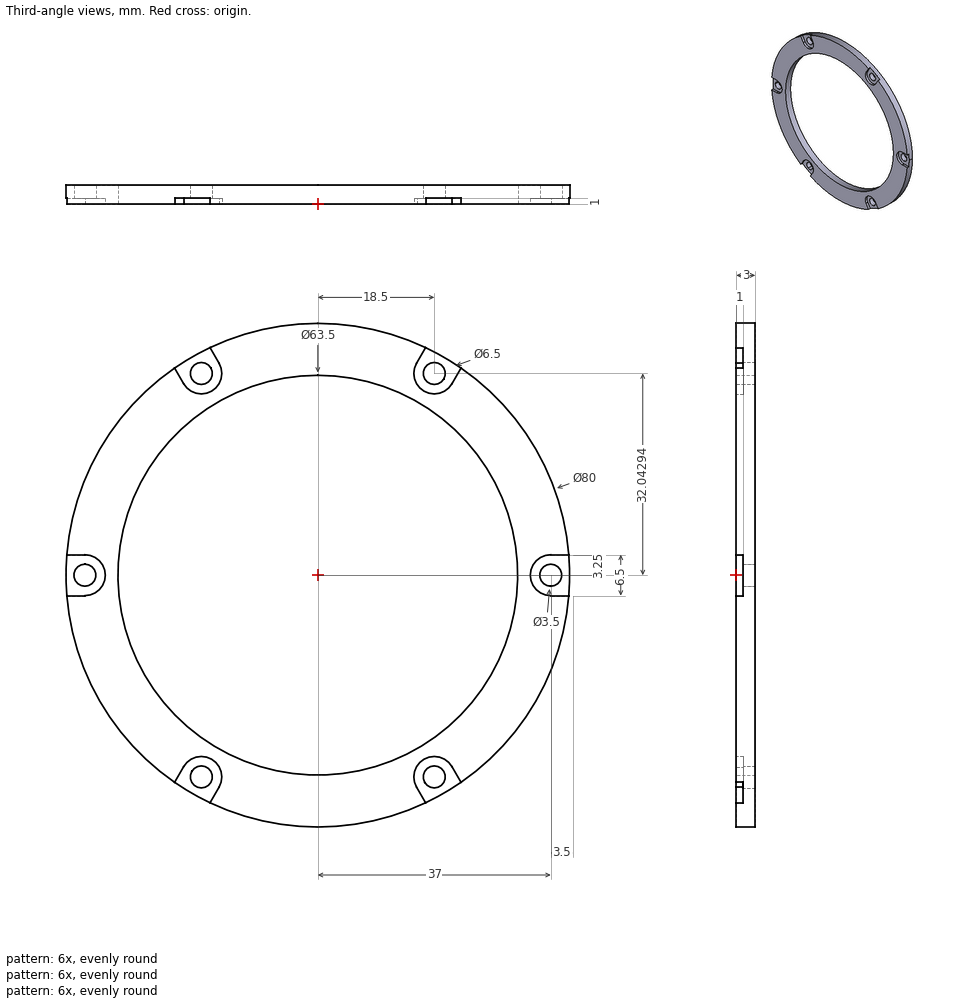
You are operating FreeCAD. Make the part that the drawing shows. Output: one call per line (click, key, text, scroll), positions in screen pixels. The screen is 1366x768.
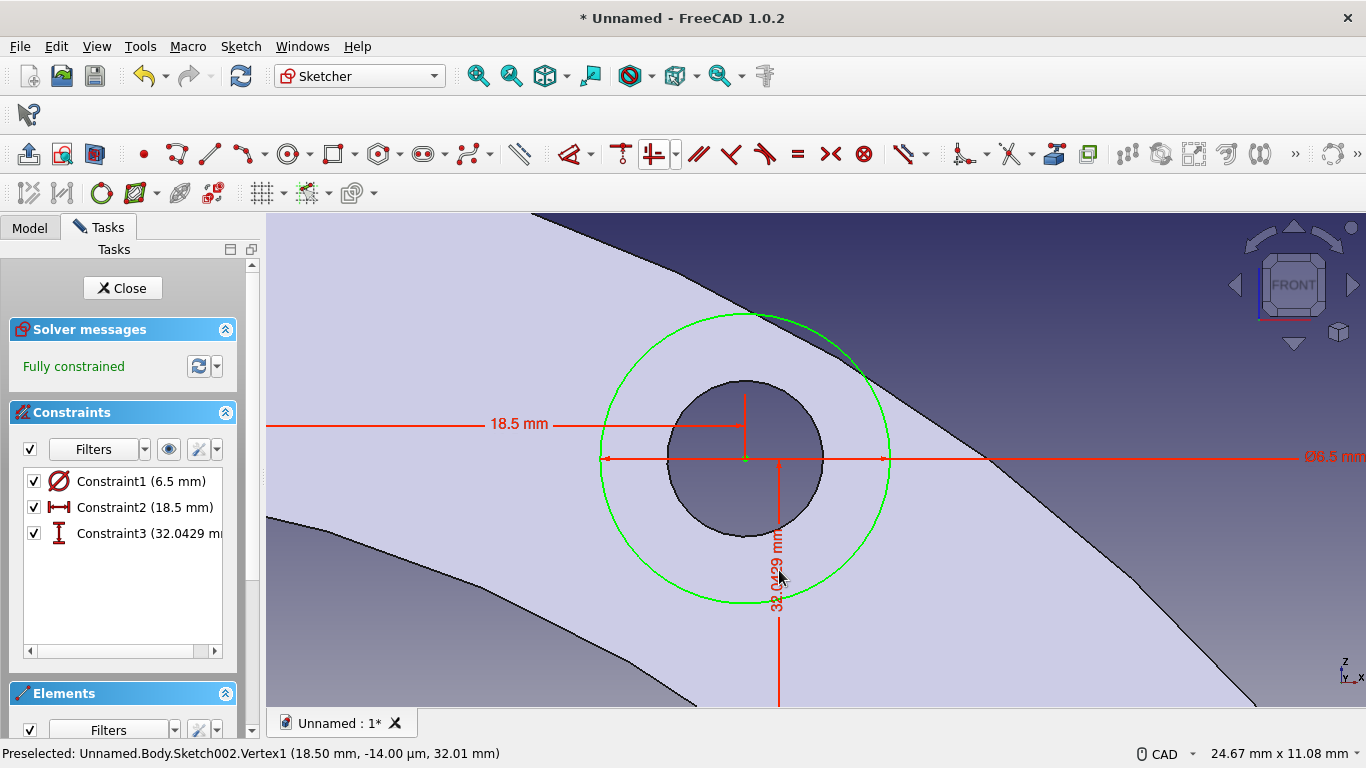
click(123, 288)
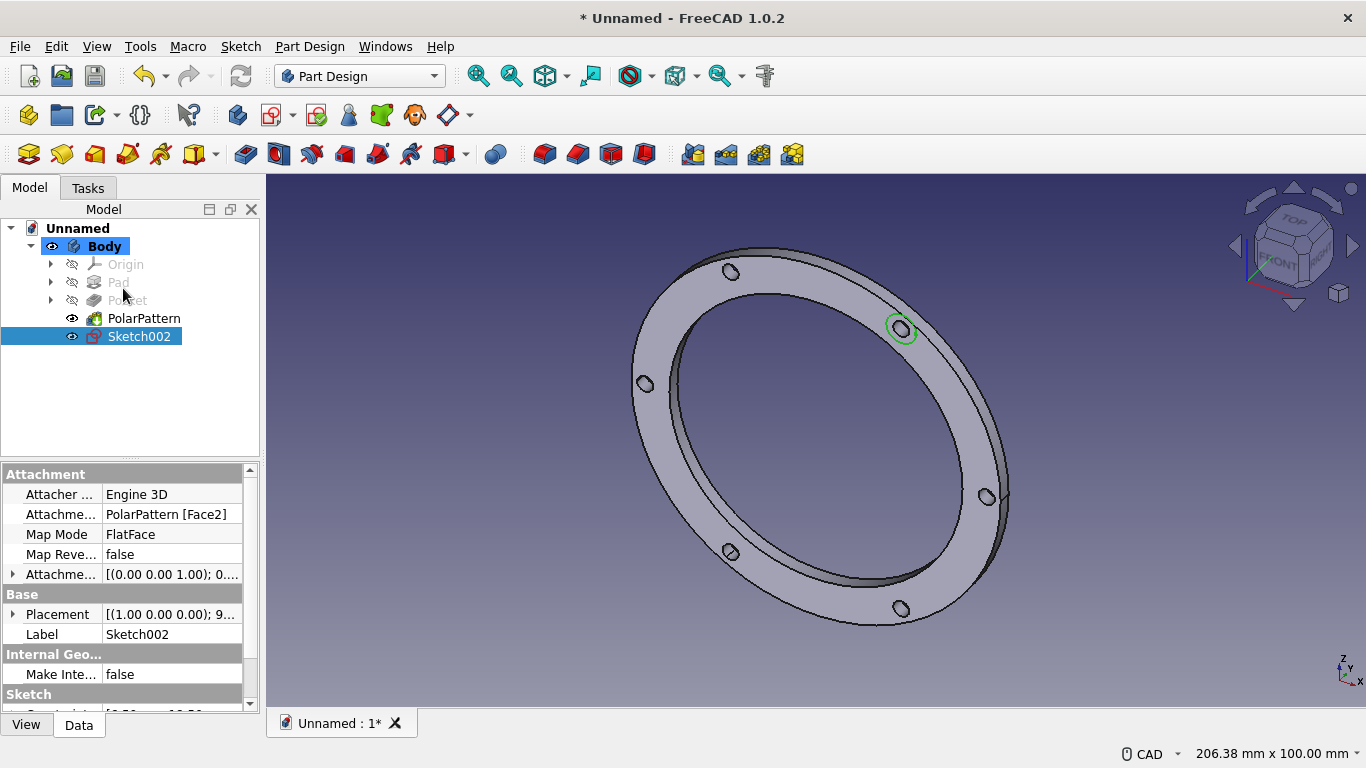
click(246, 154)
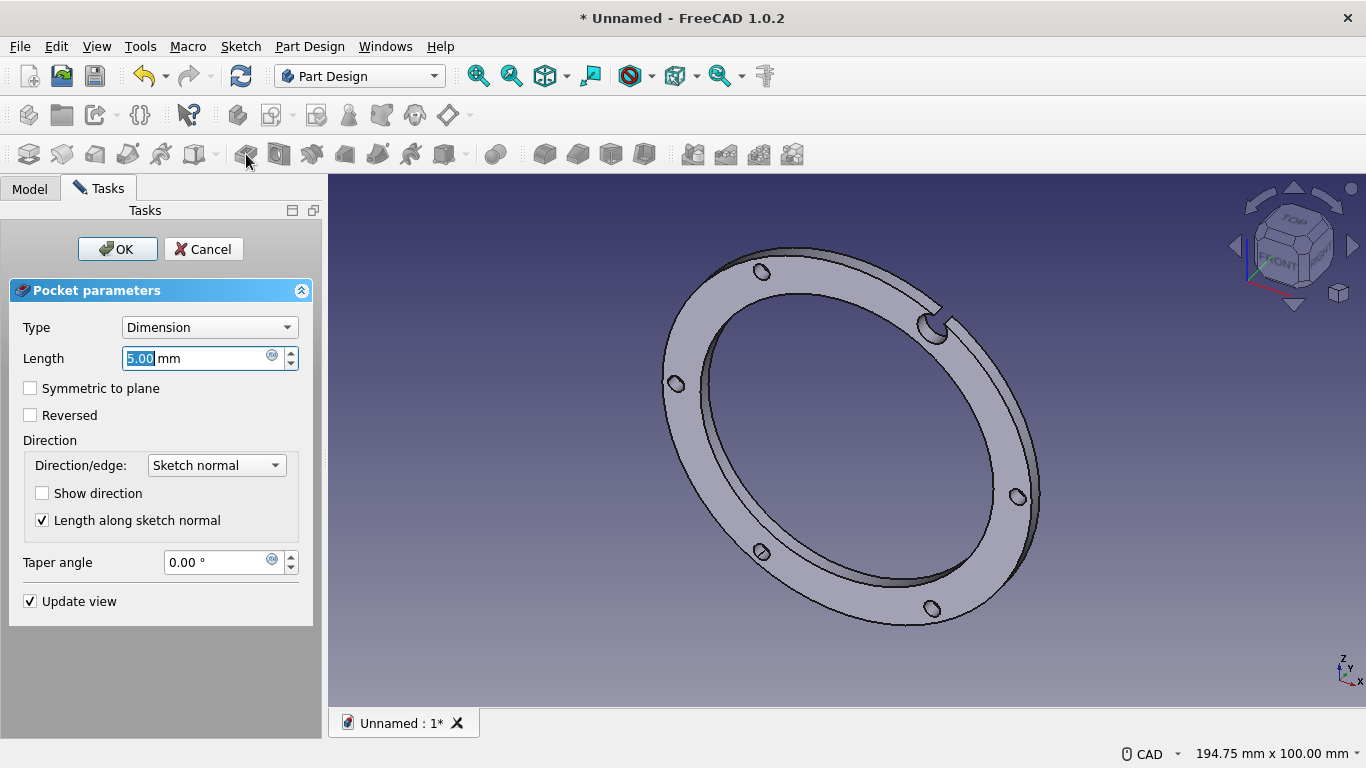
text(1)
key(Tab)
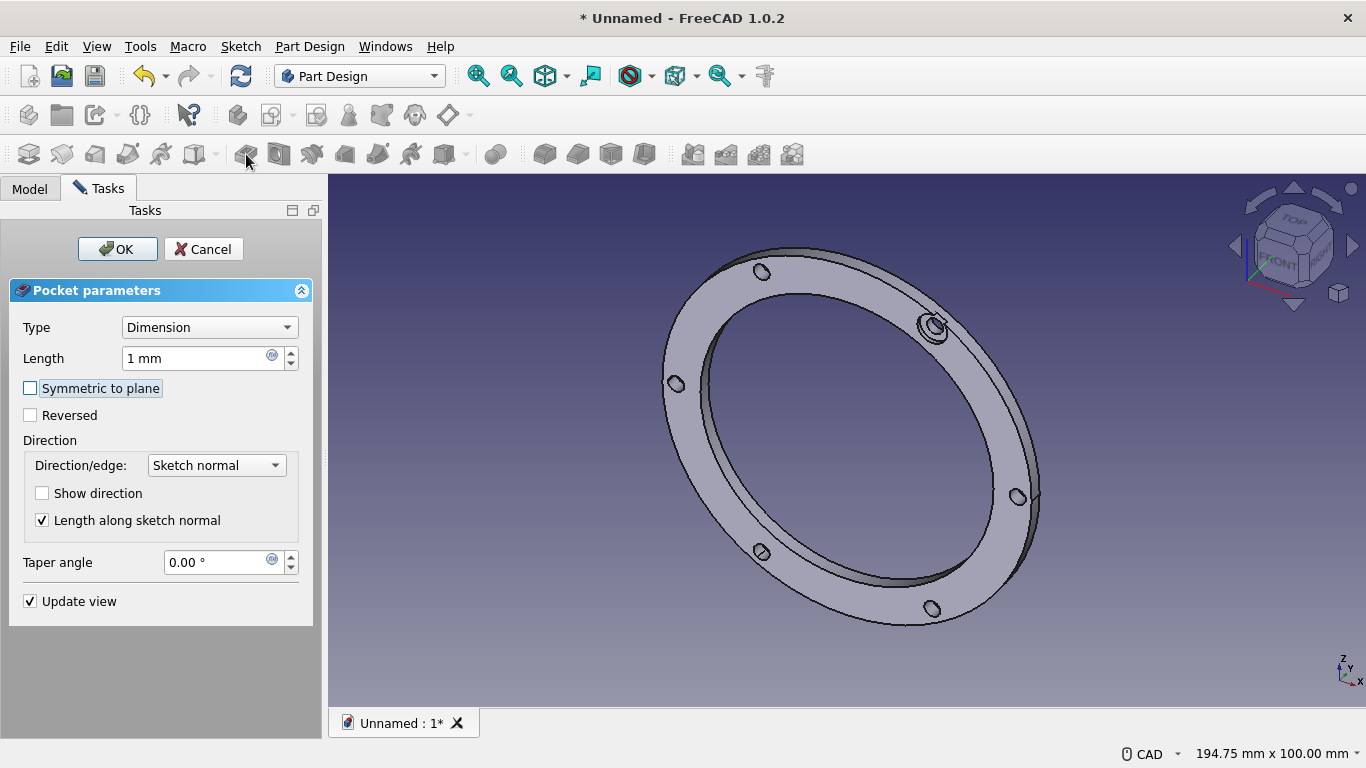
click(118, 249)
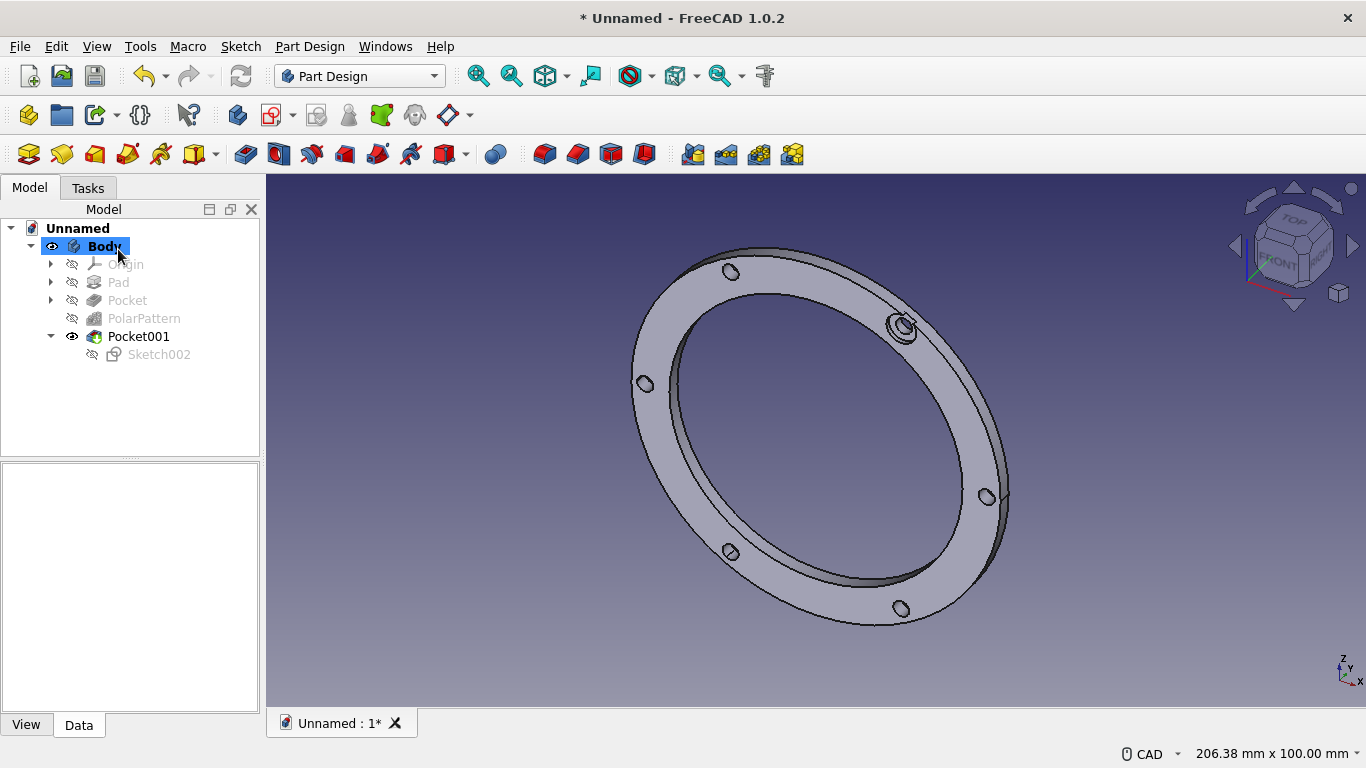
click(117, 336)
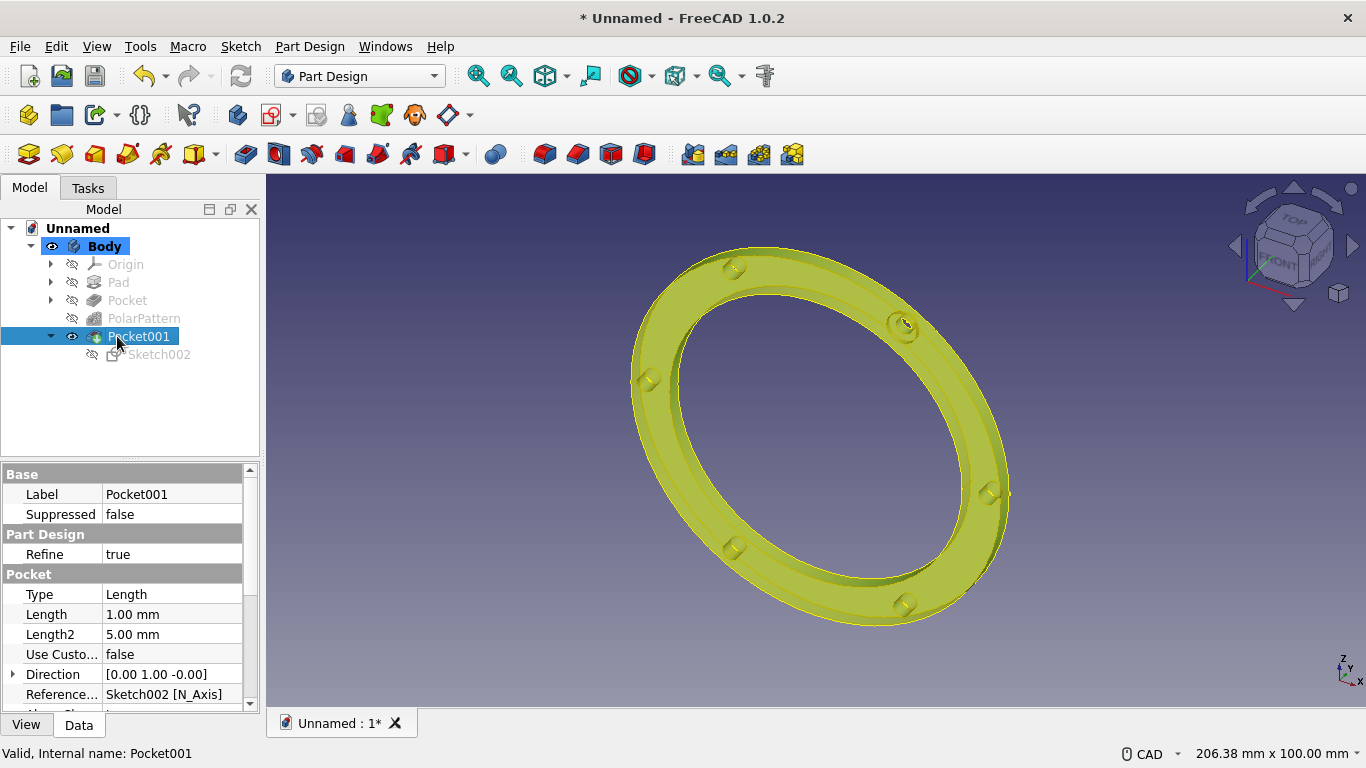
click(759, 154)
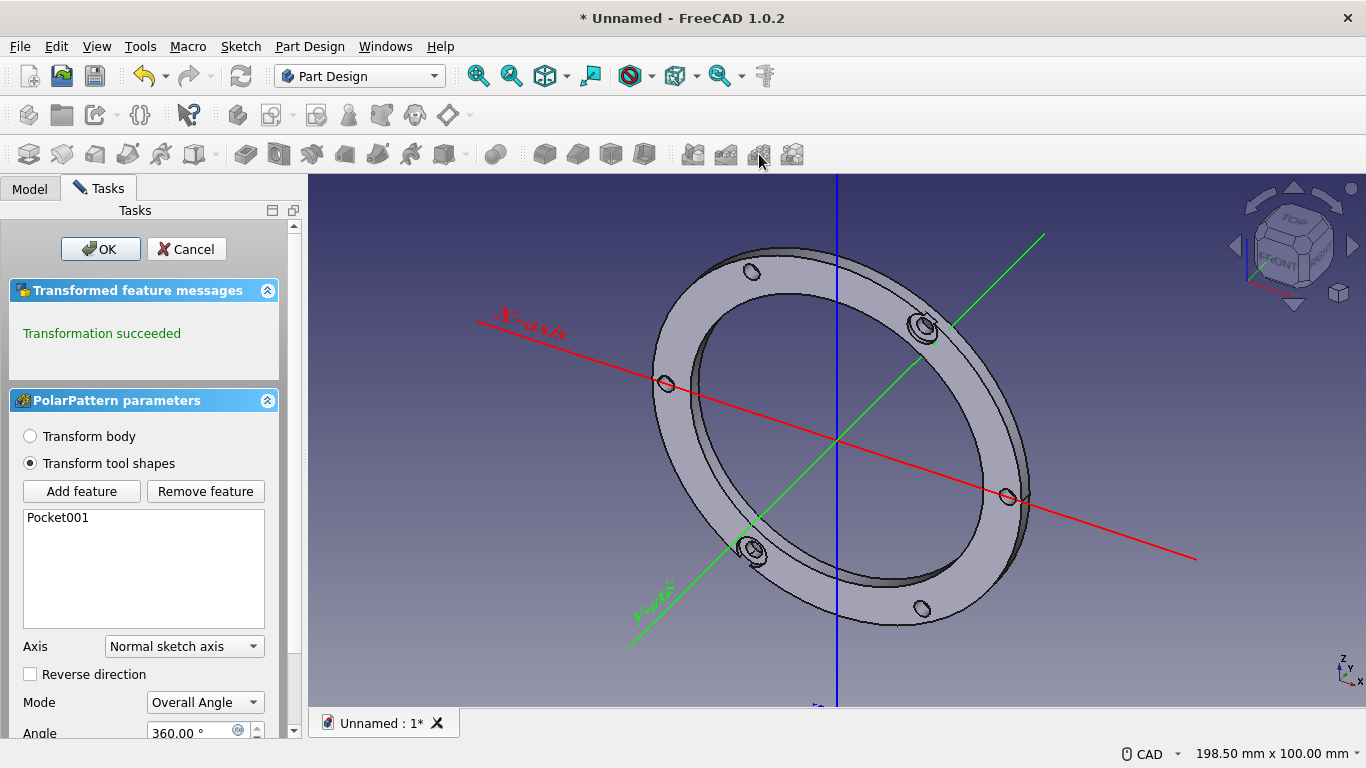
click(185, 646)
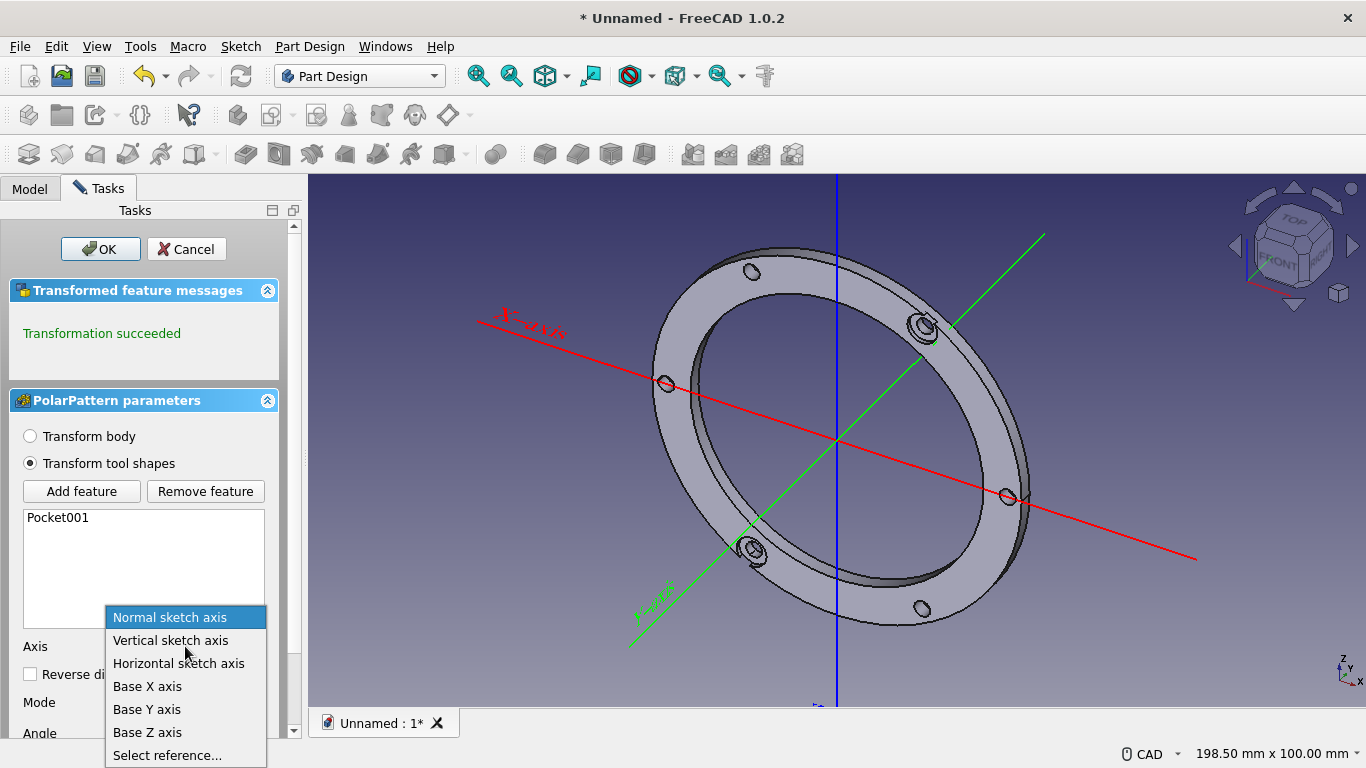
click(184, 710)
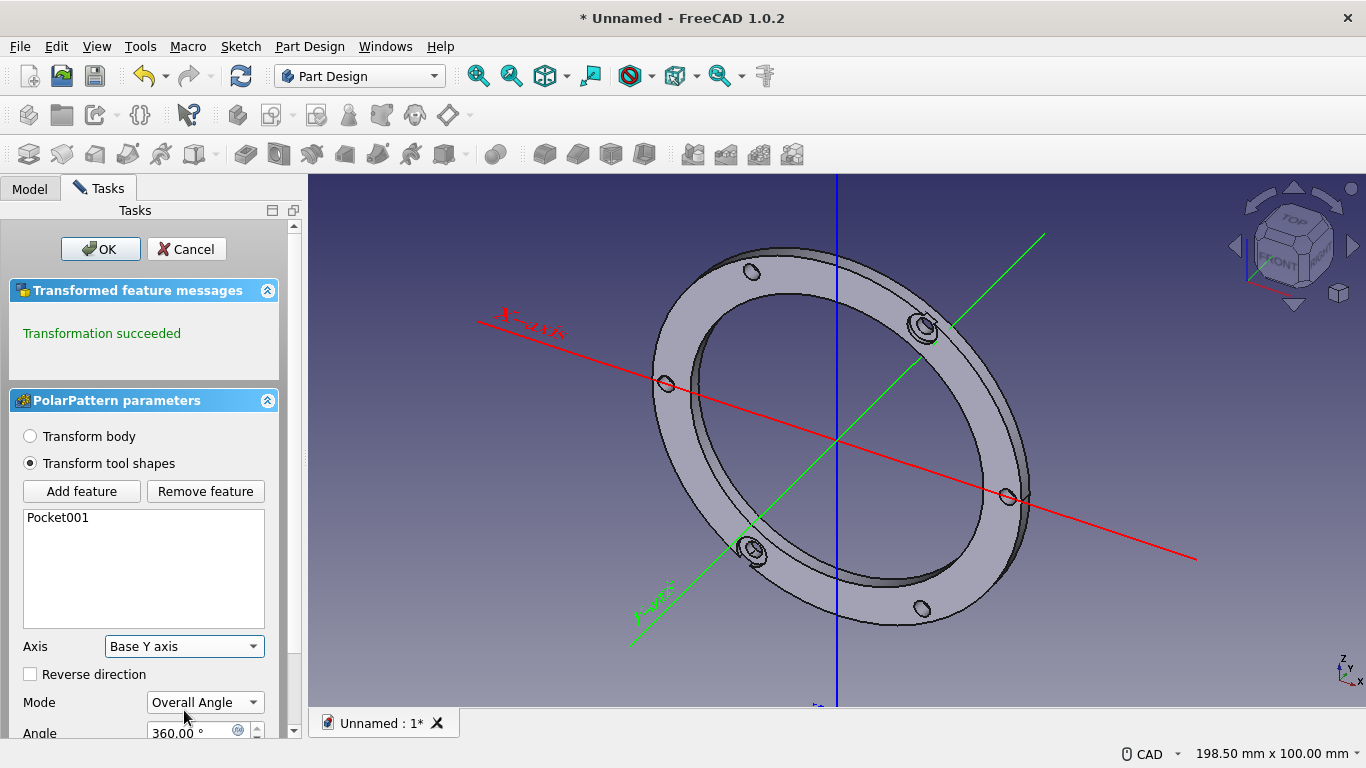
scroll(294, 479, down, 2)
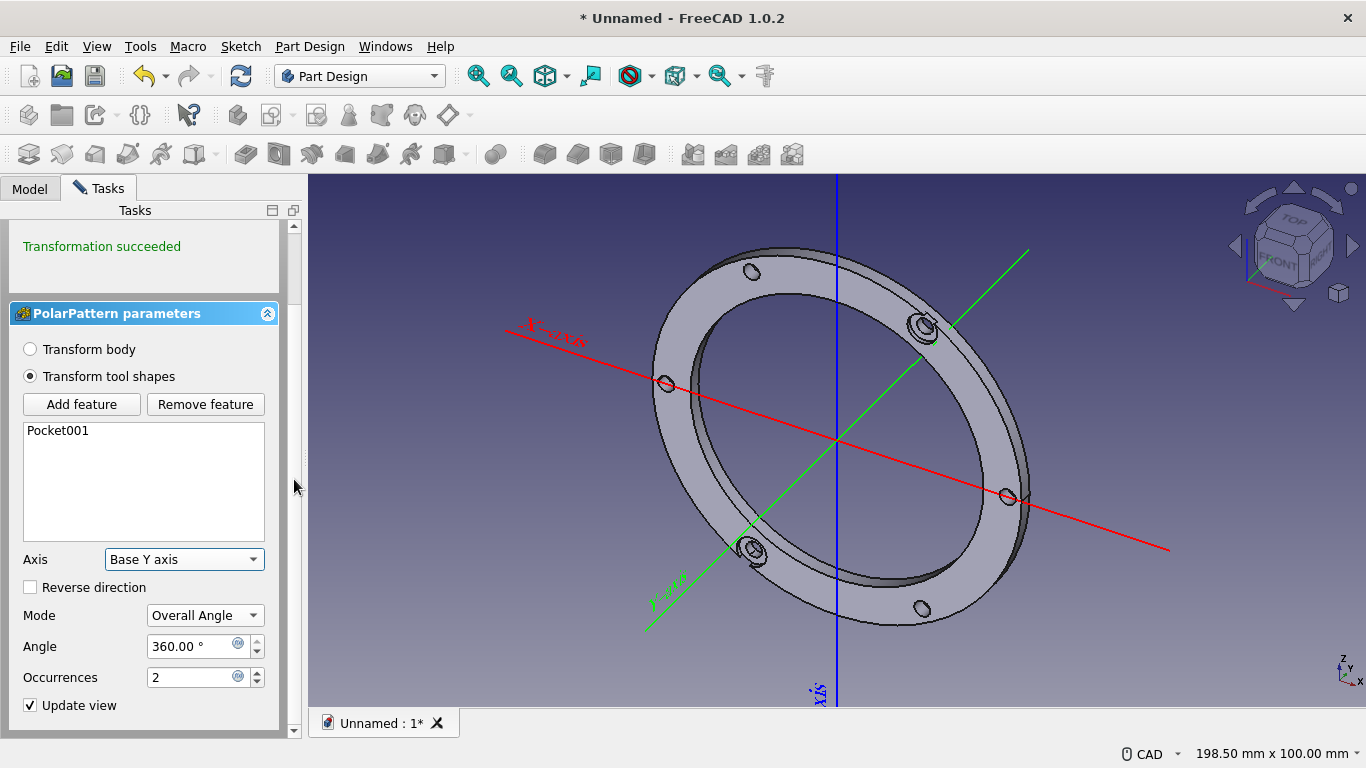
triple_click(199, 678)